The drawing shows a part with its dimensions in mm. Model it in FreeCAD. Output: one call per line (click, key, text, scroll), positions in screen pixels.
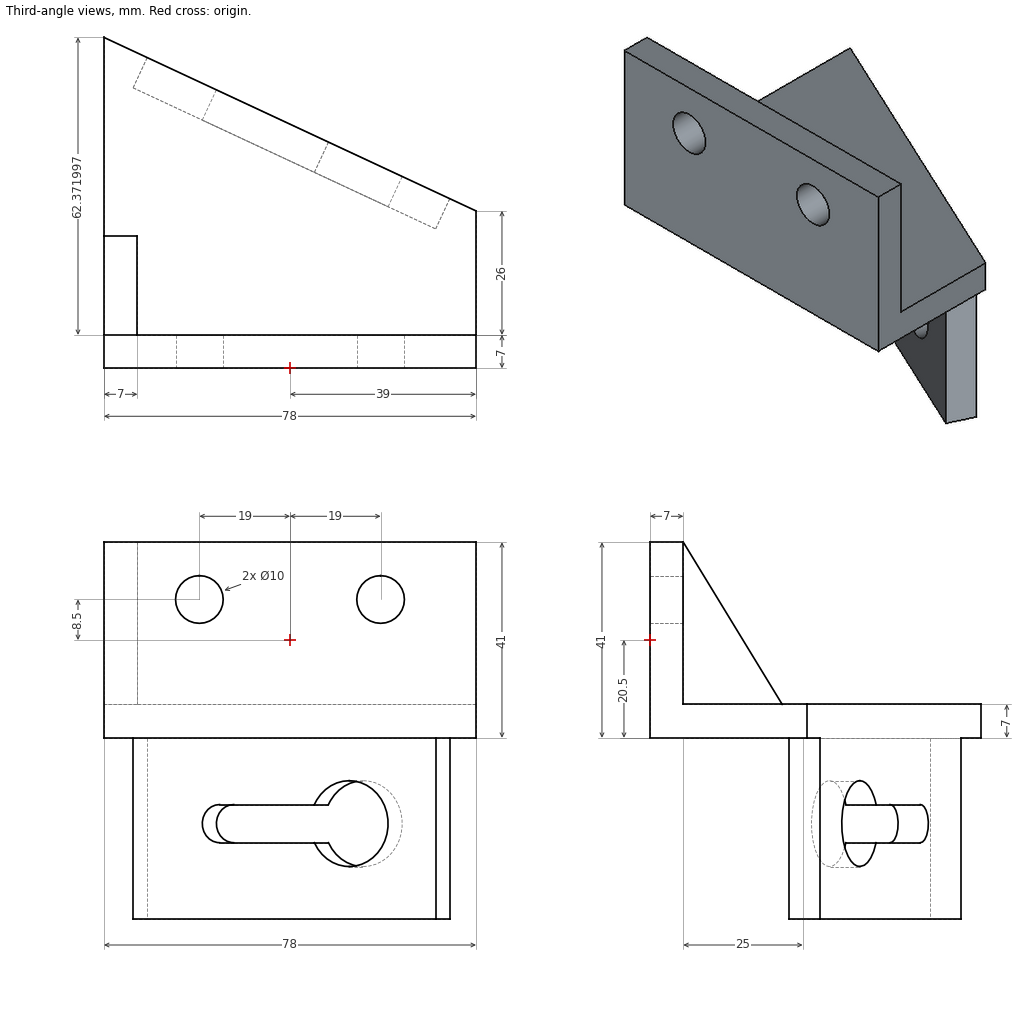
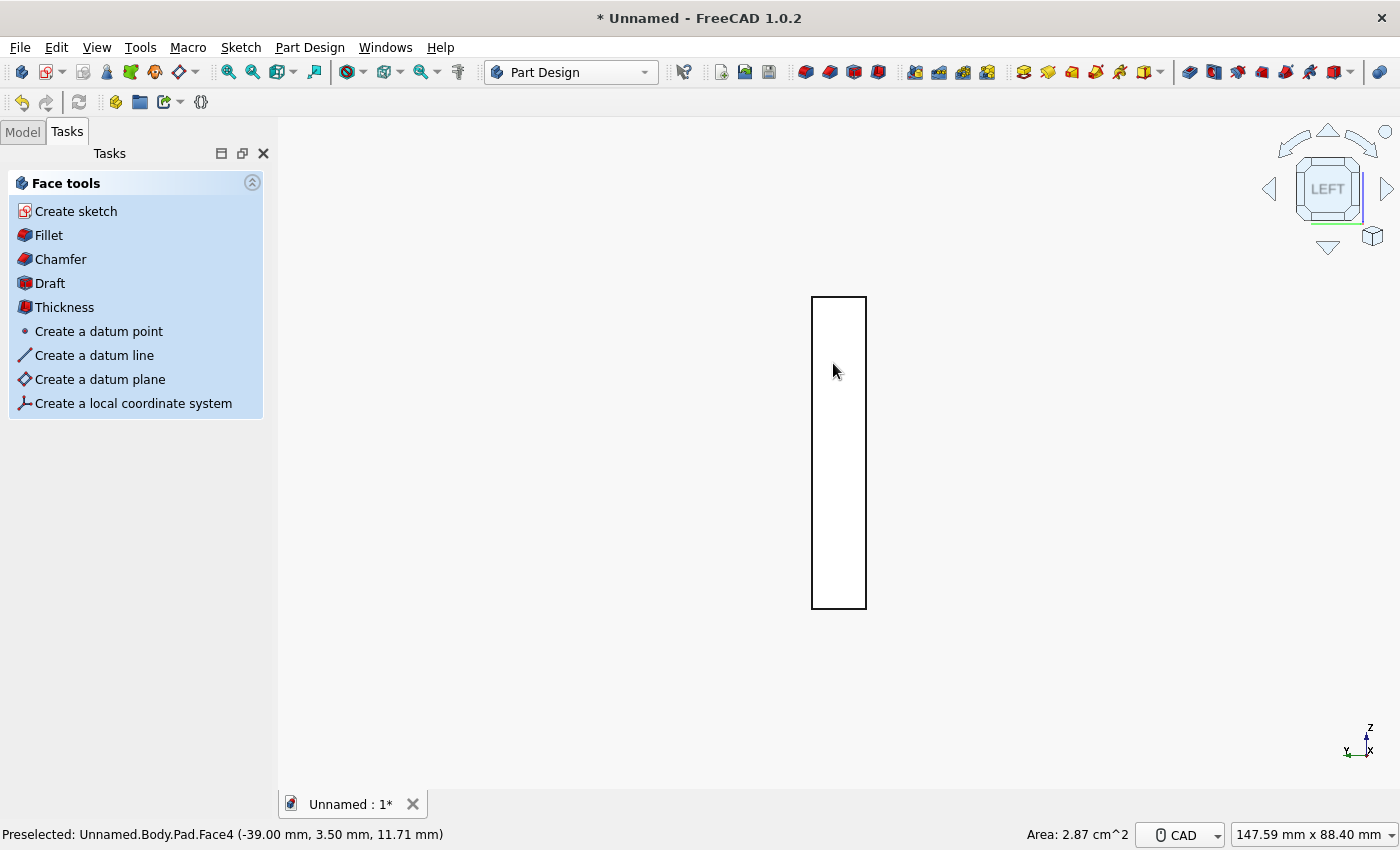
click(46, 72)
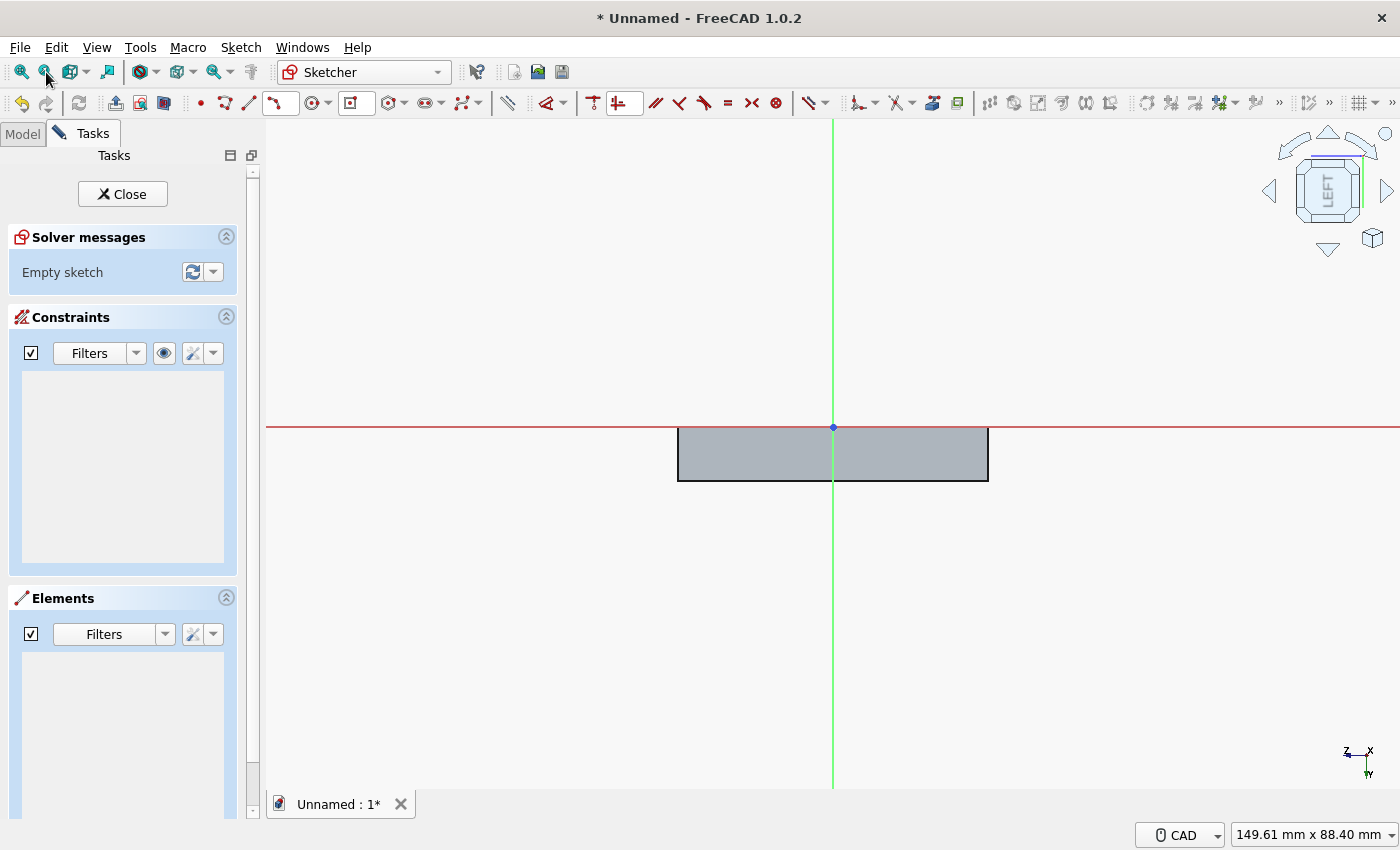
scroll(916, 664, up, 3)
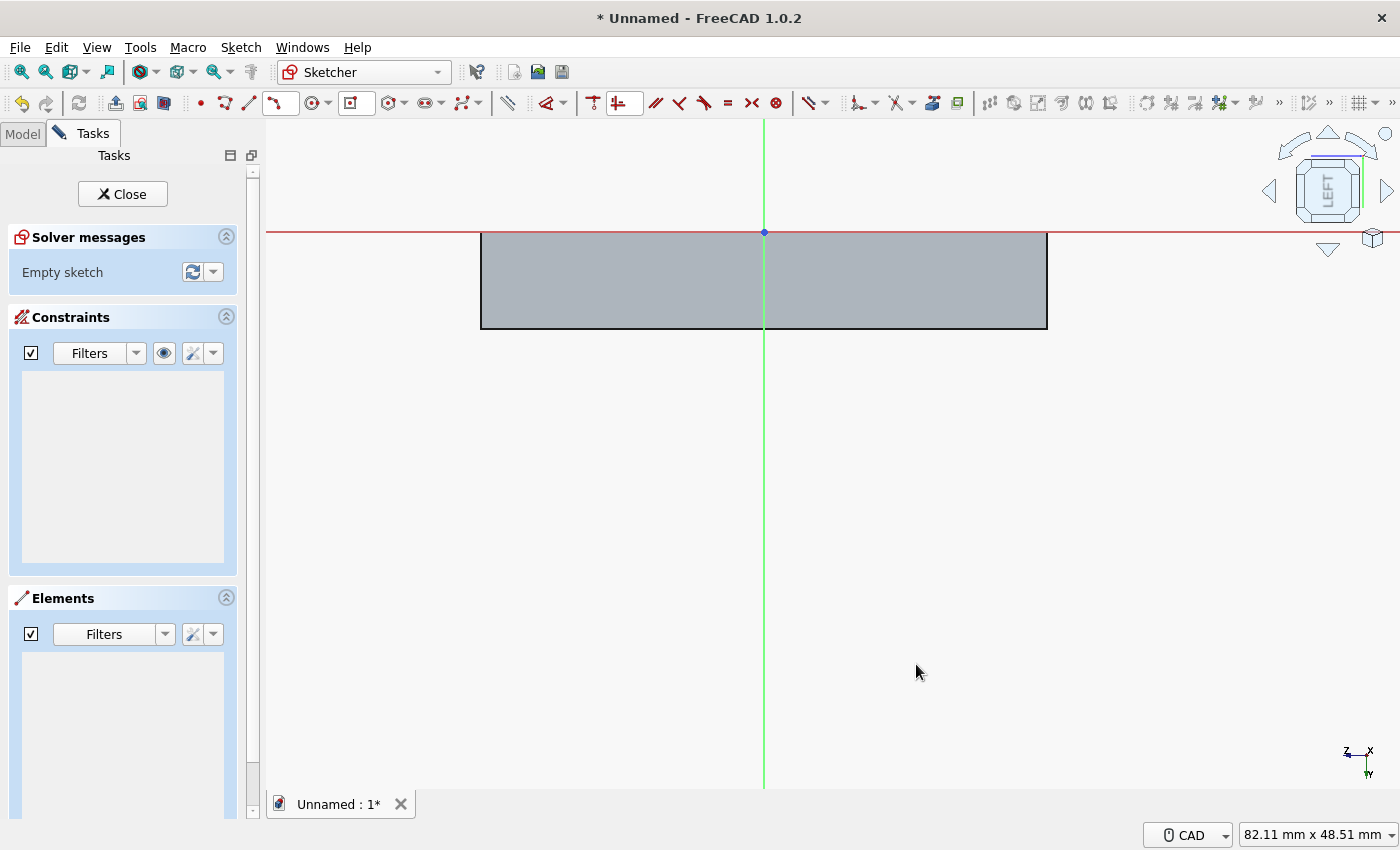
key(g)
key(m)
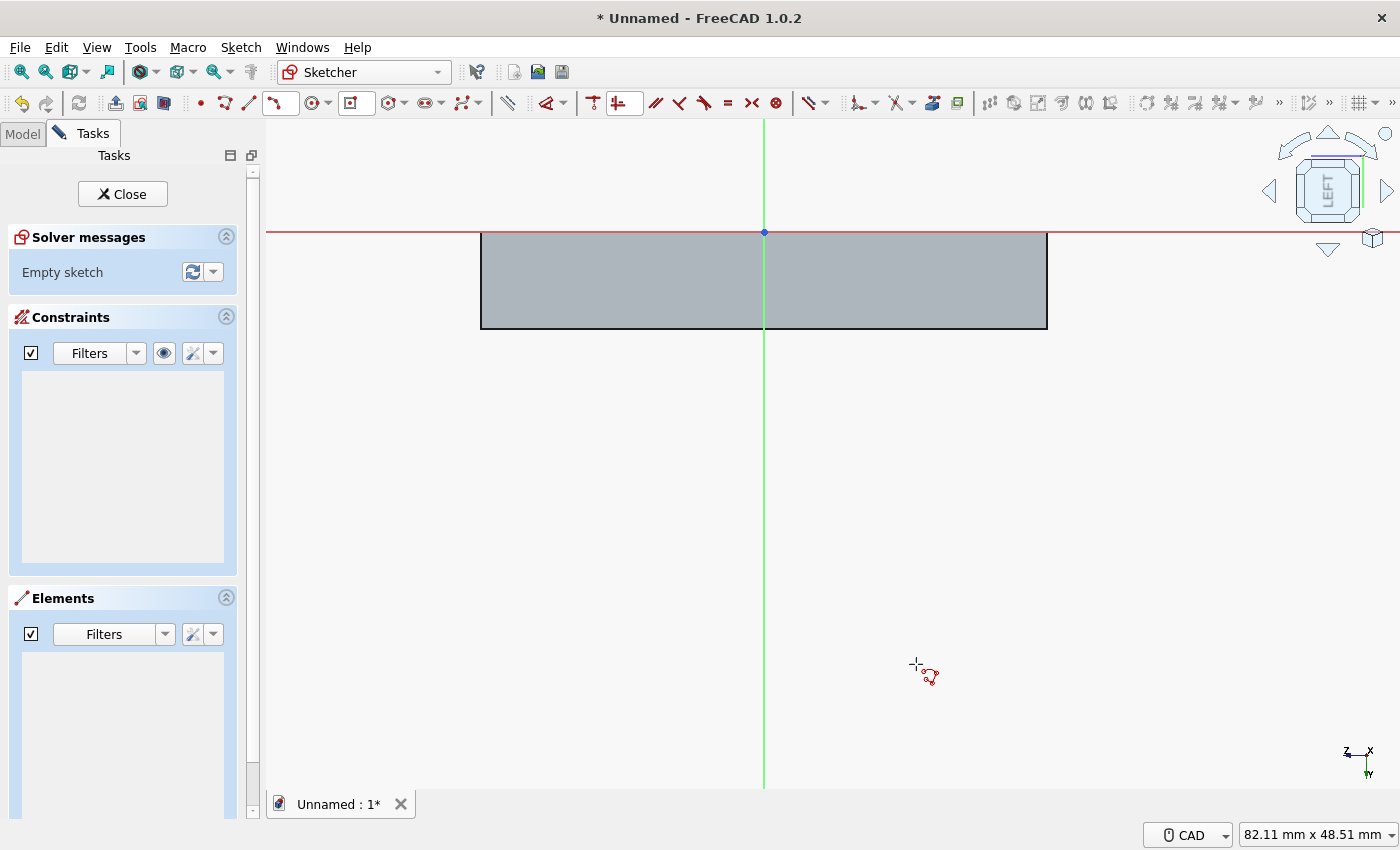
click(1047, 329)
click(481, 329)
click(1047, 674)
click(1047, 330)
key(Escape)
key(Escape)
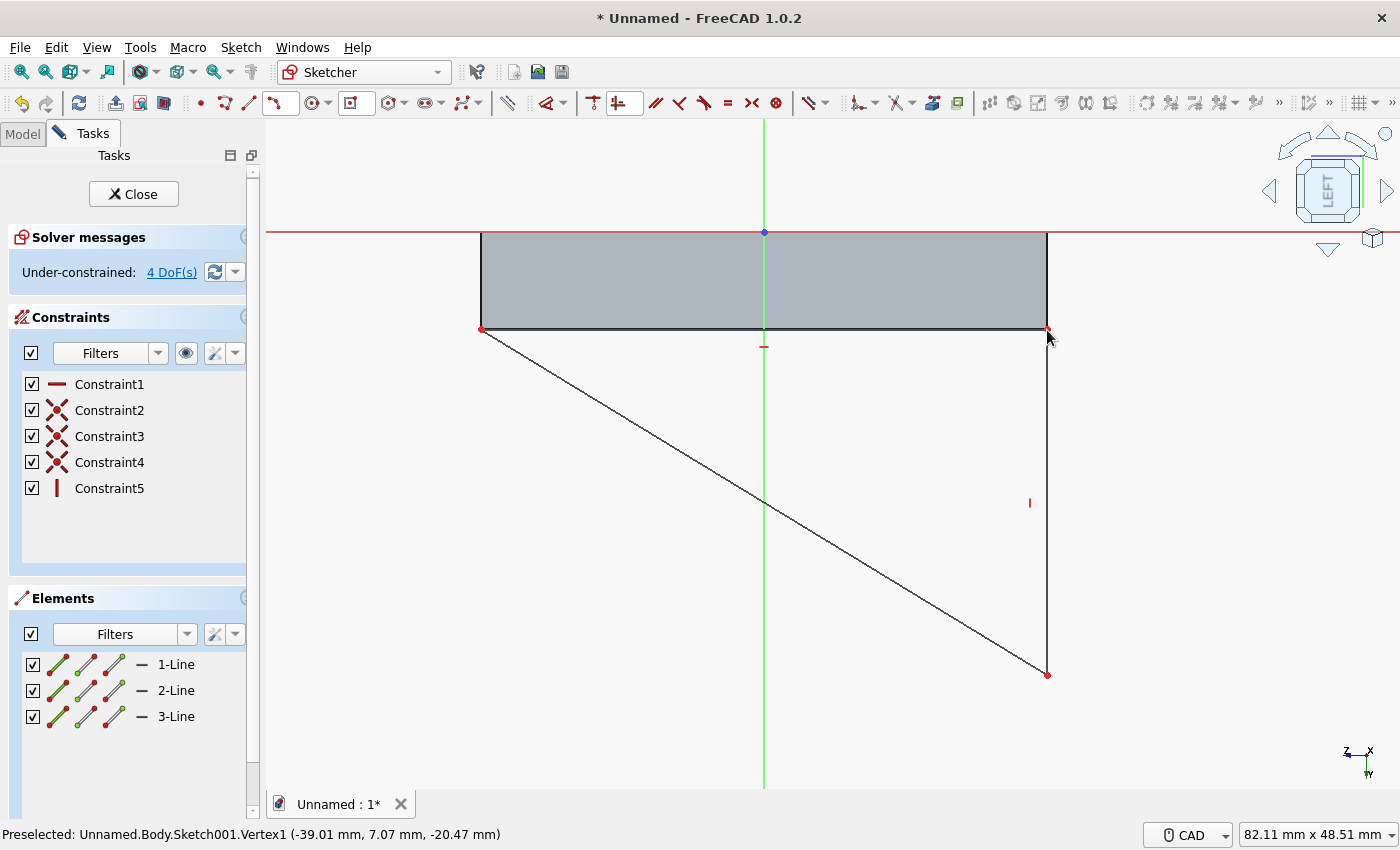
click(546, 104)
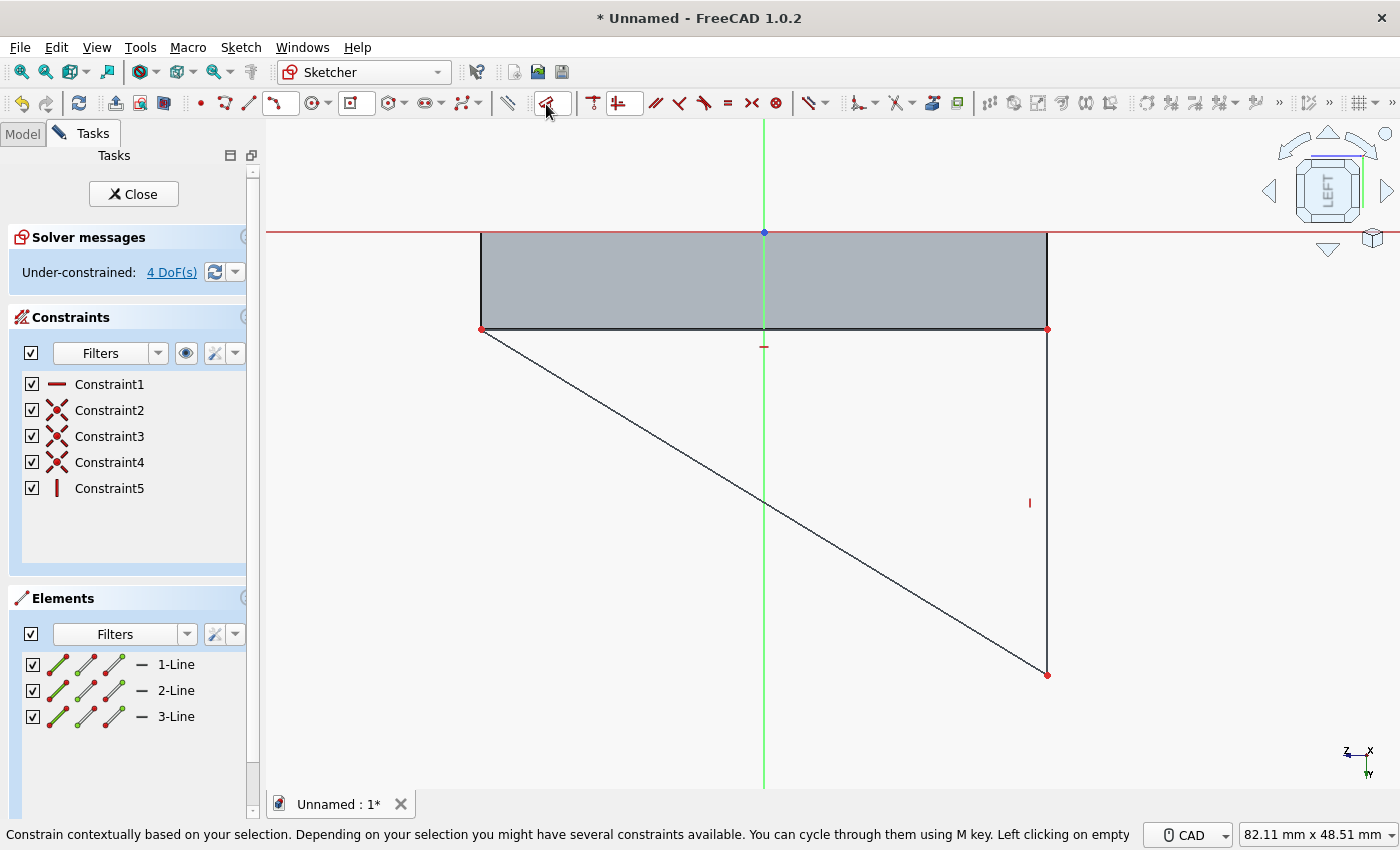
click(877, 330)
click(634, 296)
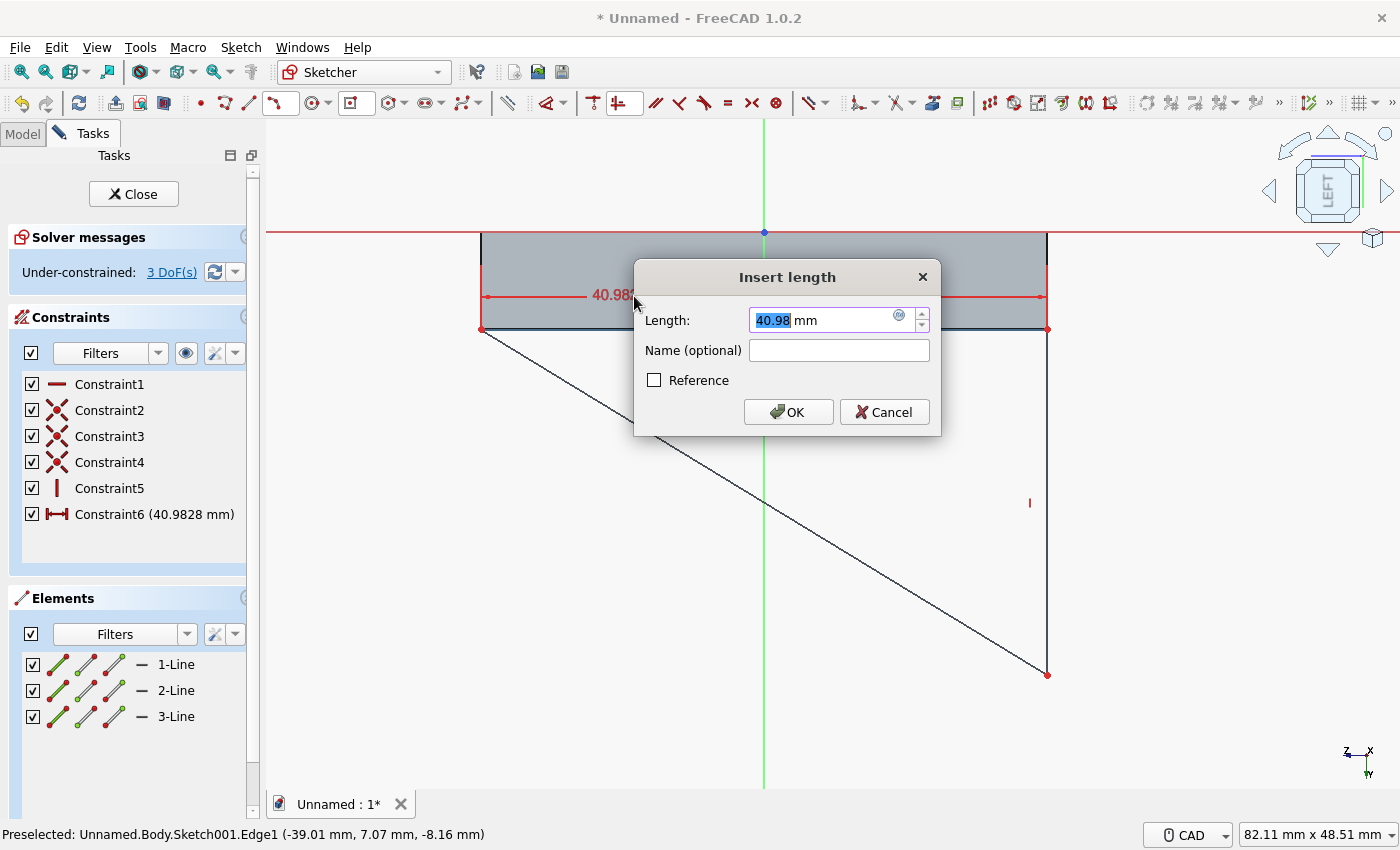
text(41)
key(Return)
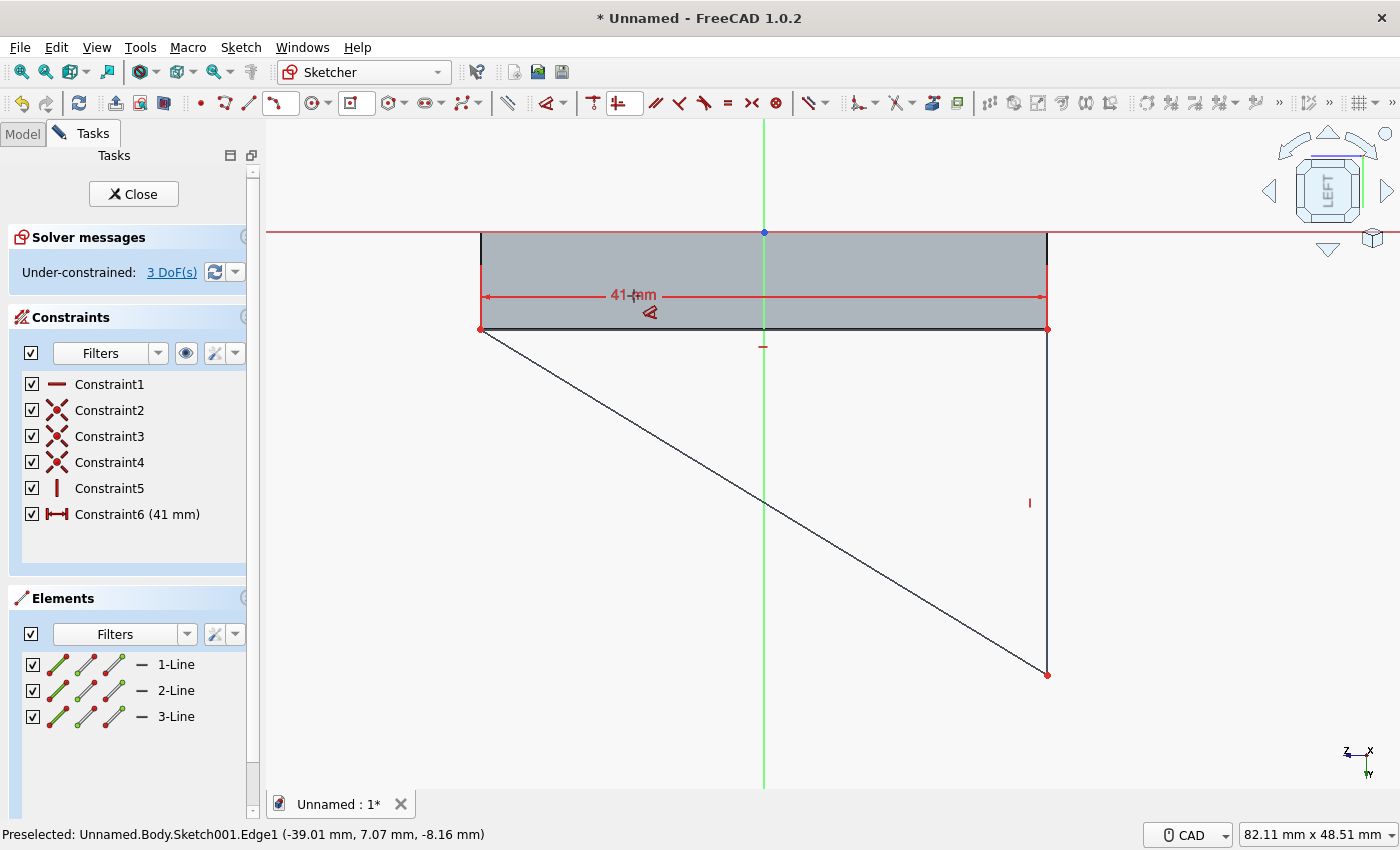
click(1047, 572)
click(1081, 503)